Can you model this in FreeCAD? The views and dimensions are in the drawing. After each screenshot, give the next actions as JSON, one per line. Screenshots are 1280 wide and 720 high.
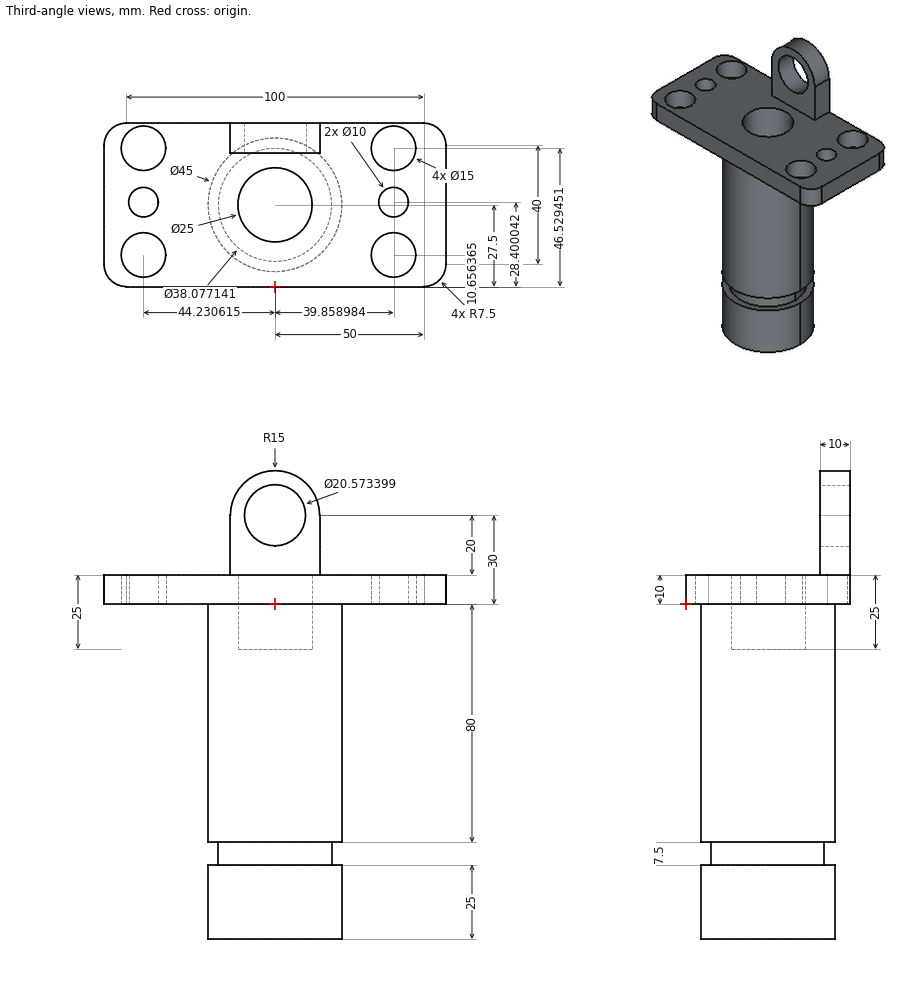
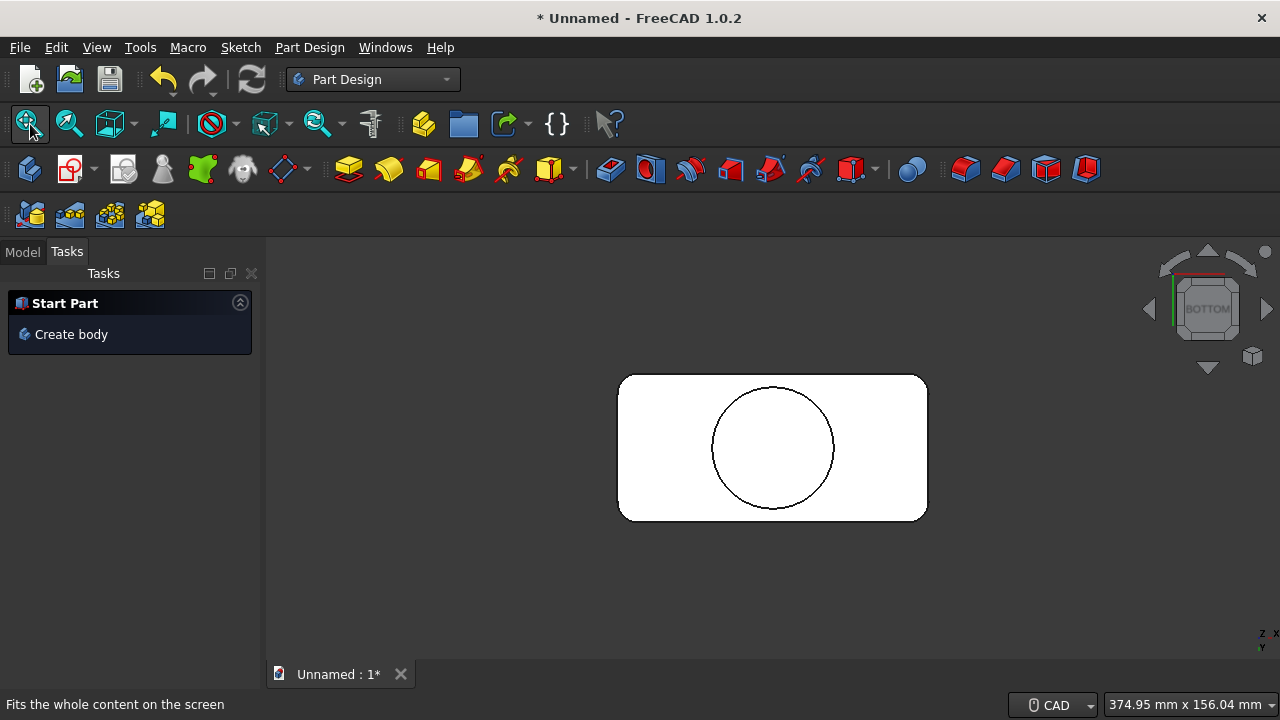
{"action": "left_click", "coordinate": [773, 447]}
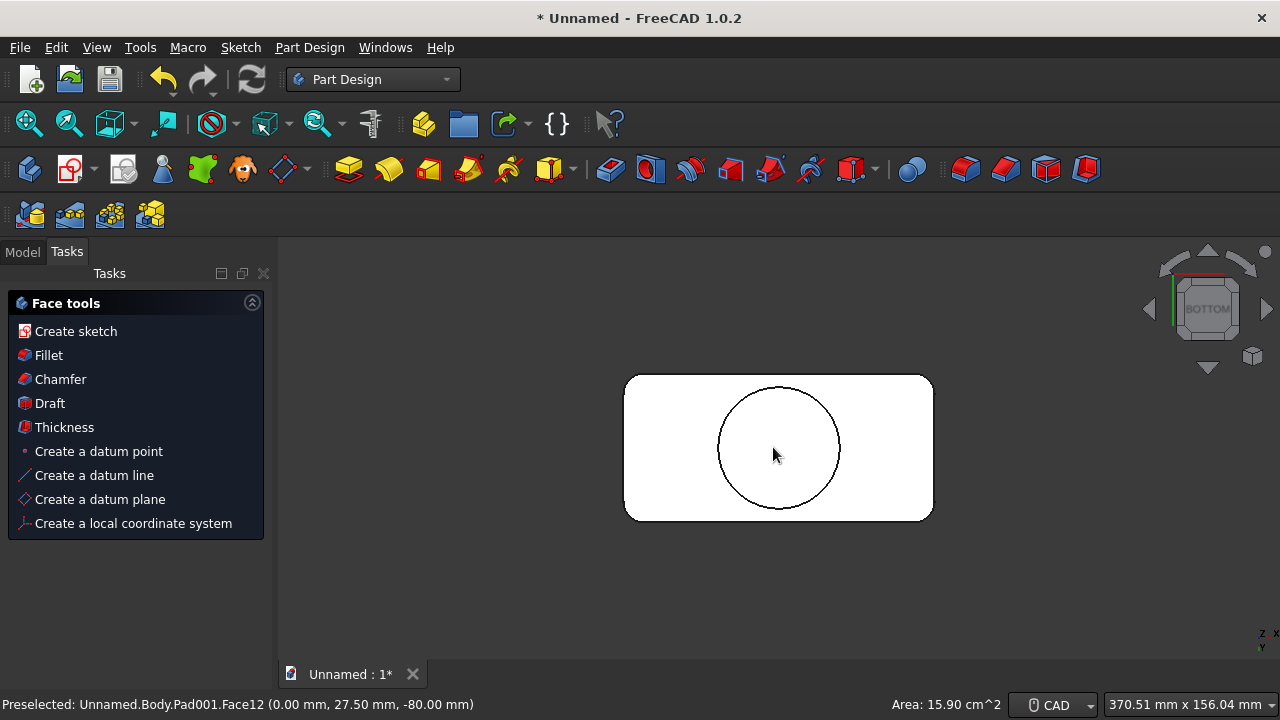
{"action": "left_click", "coordinate": [70, 170]}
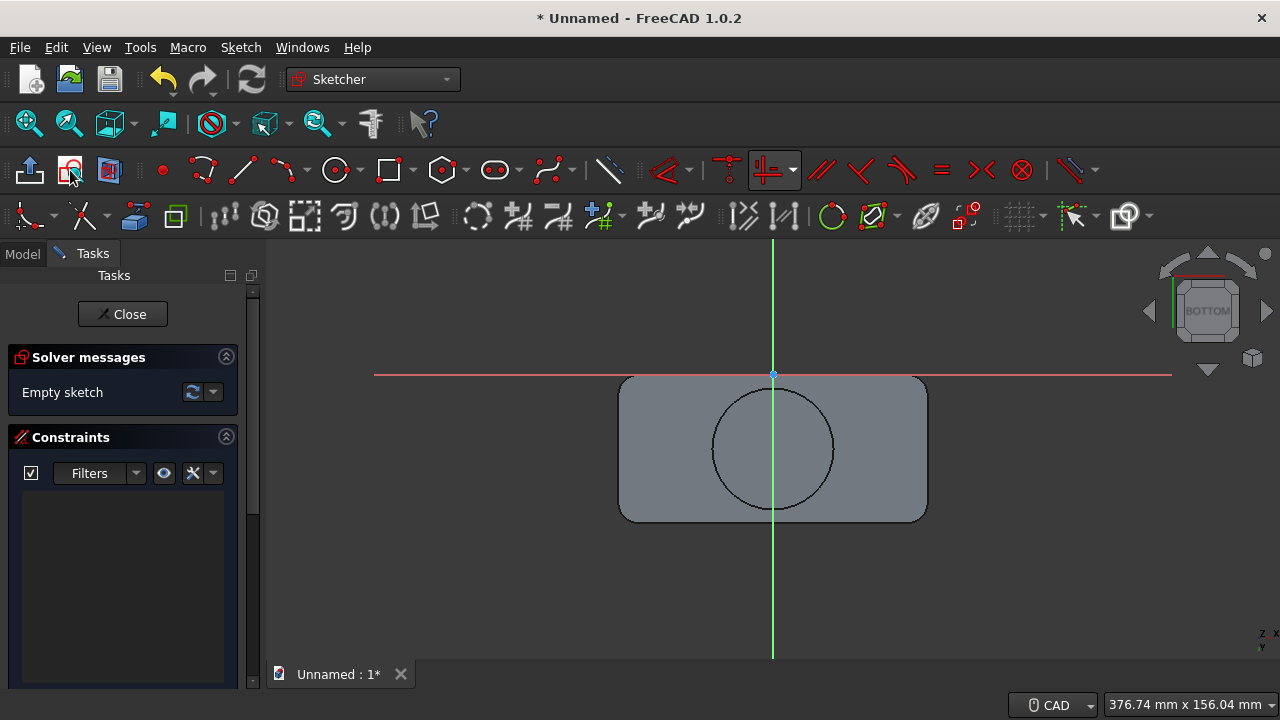
{"action": "scroll", "coordinate": [829, 428], "scroll_direction": "up", "scroll_amount": 4}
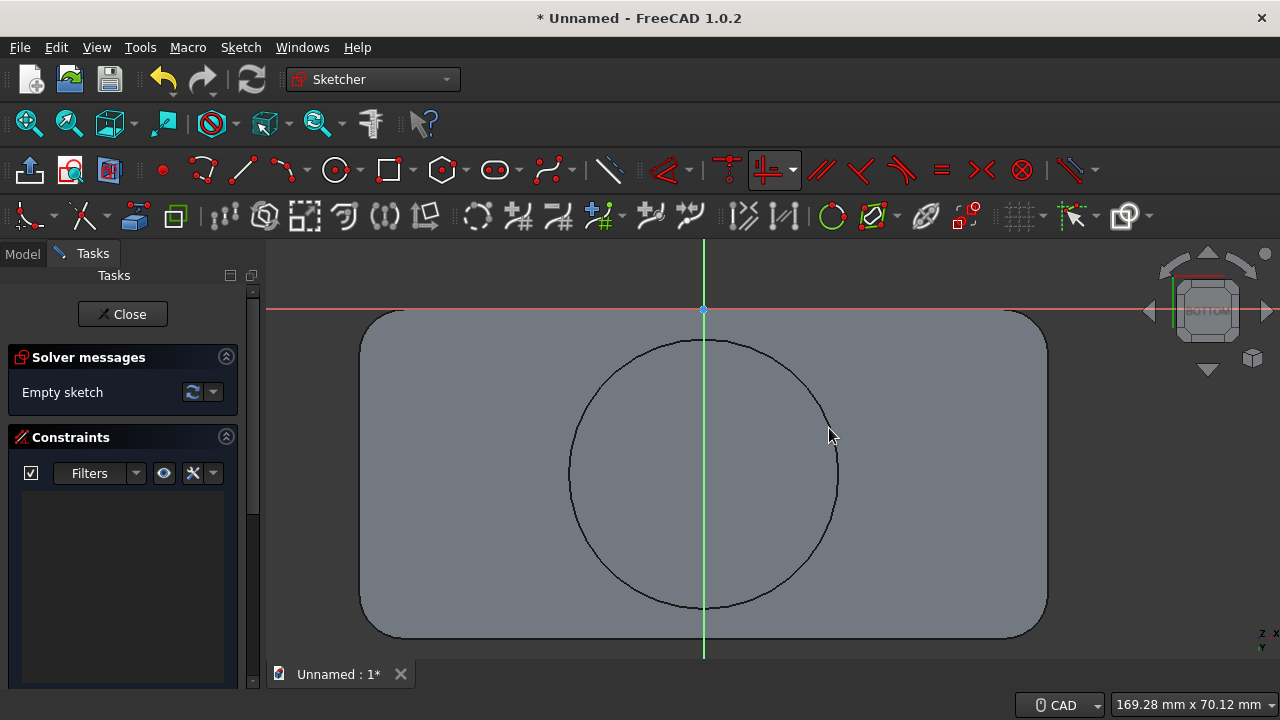
{"action": "left_click", "coordinate": [336, 170]}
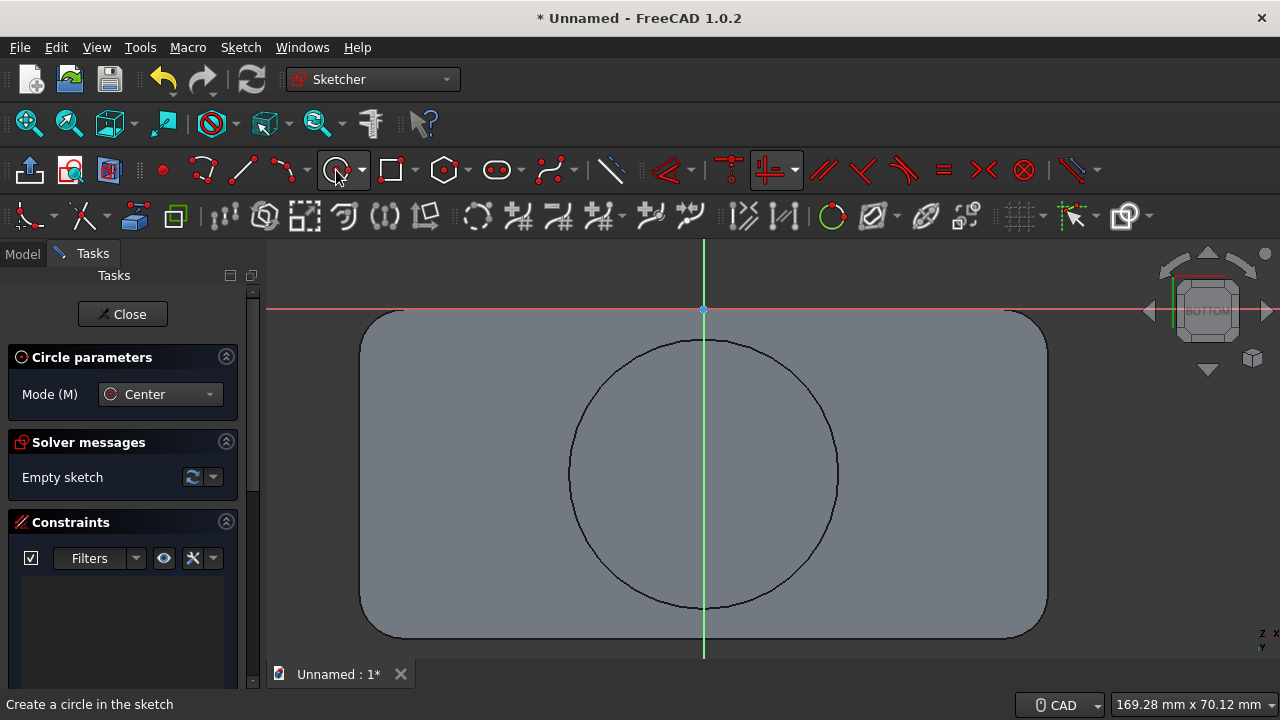
{"action": "left_click", "coordinate": [704, 474]}
{"action": "left_click", "coordinate": [784, 394]}
{"action": "key", "text": "Escape"}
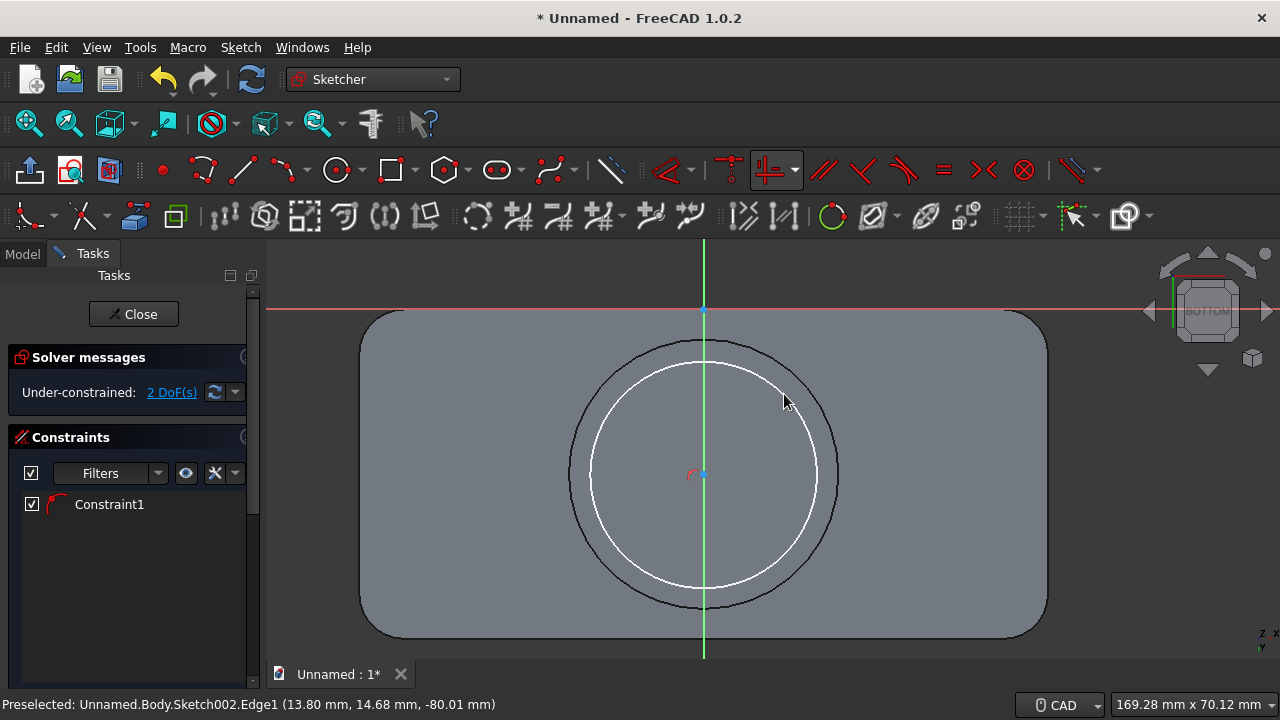
{"action": "left_click", "coordinate": [666, 170]}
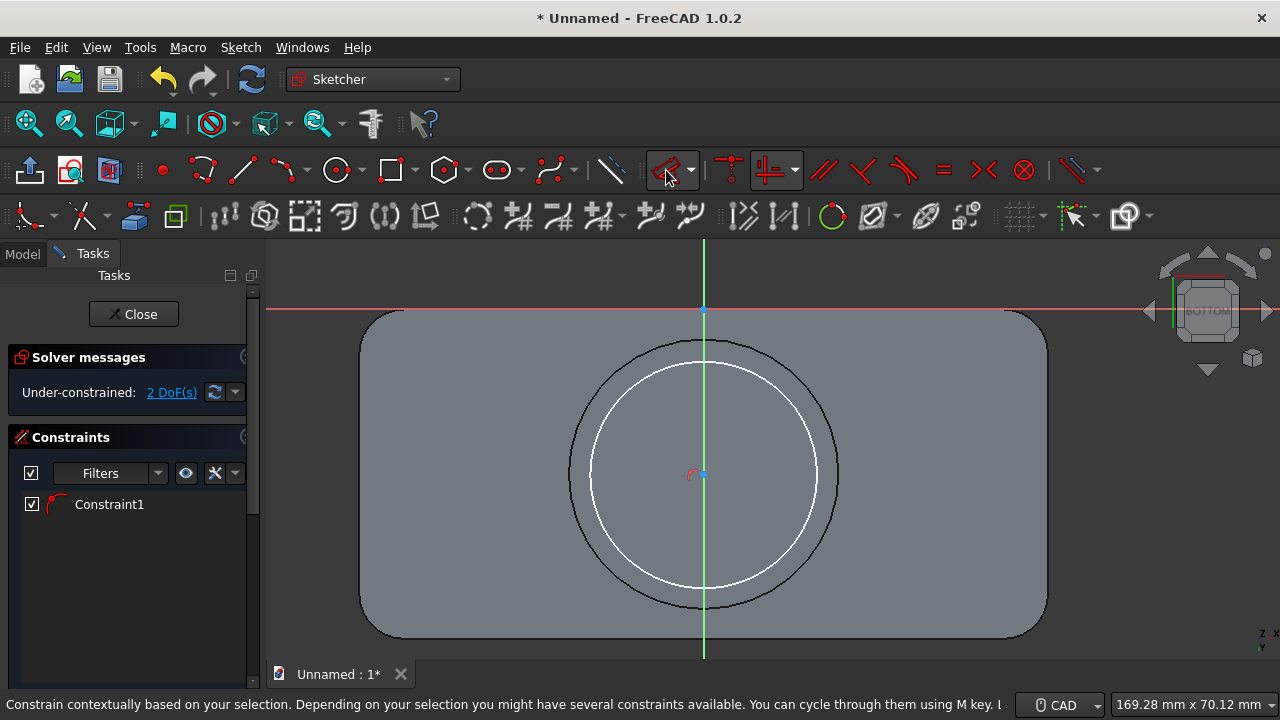
{"action": "left_click", "coordinate": [784, 395]}
{"action": "left_click", "coordinate": [807, 372]}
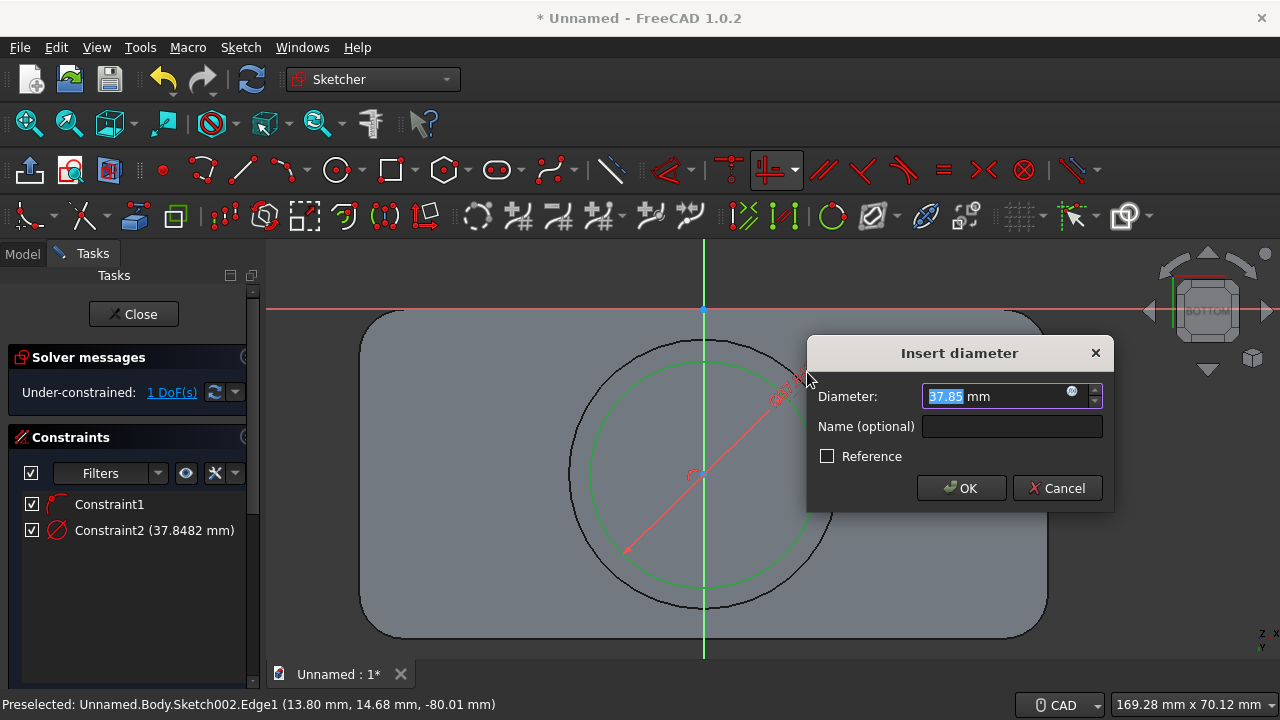
{"action": "type", "text": "38.077141"}
{"action": "key", "text": "Return"}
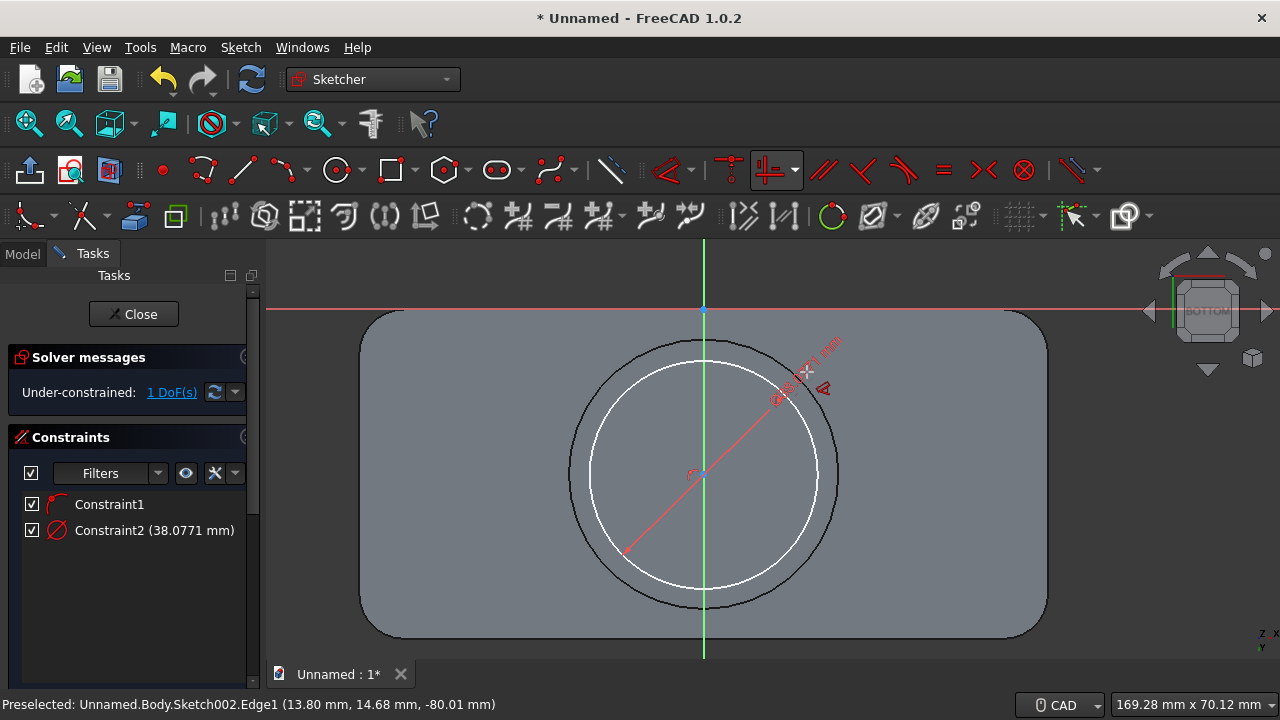
{"action": "left_click", "coordinate": [704, 475]}
{"action": "left_click", "coordinate": [738, 430]}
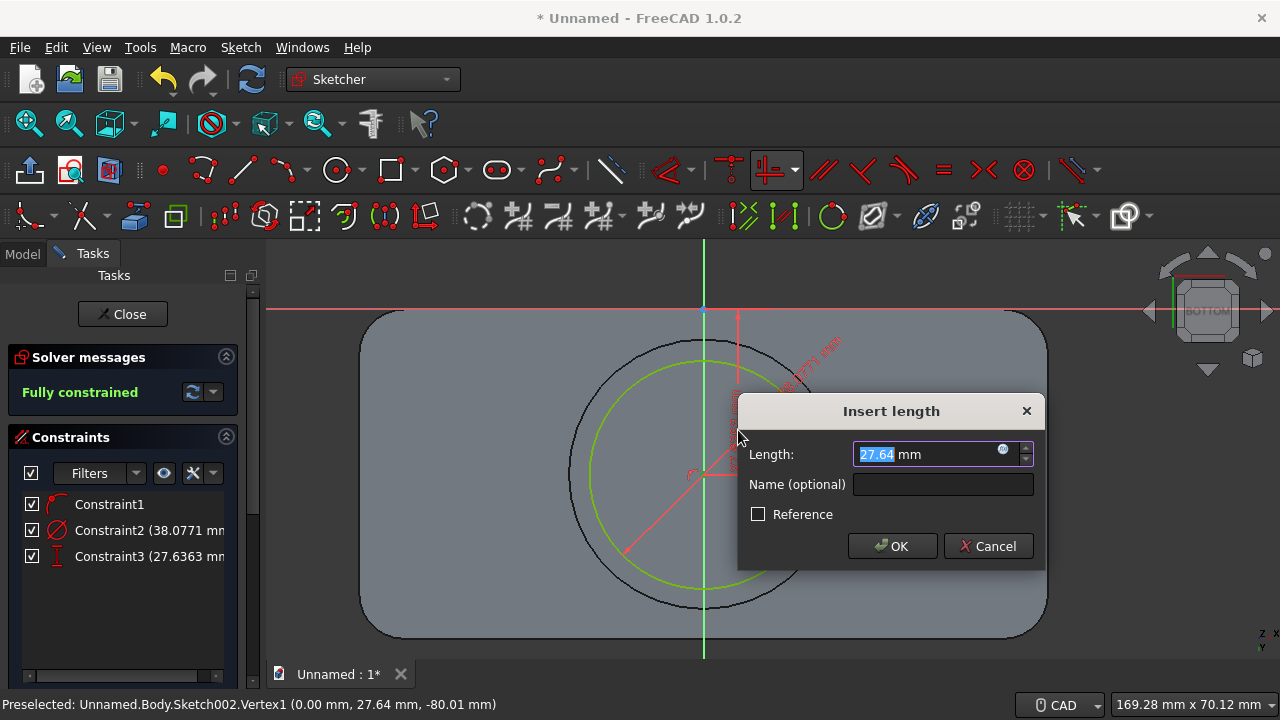
{"action": "type", "text": "27.5"}
{"action": "key", "text": "Return"}
{"action": "key", "text": "Escape"}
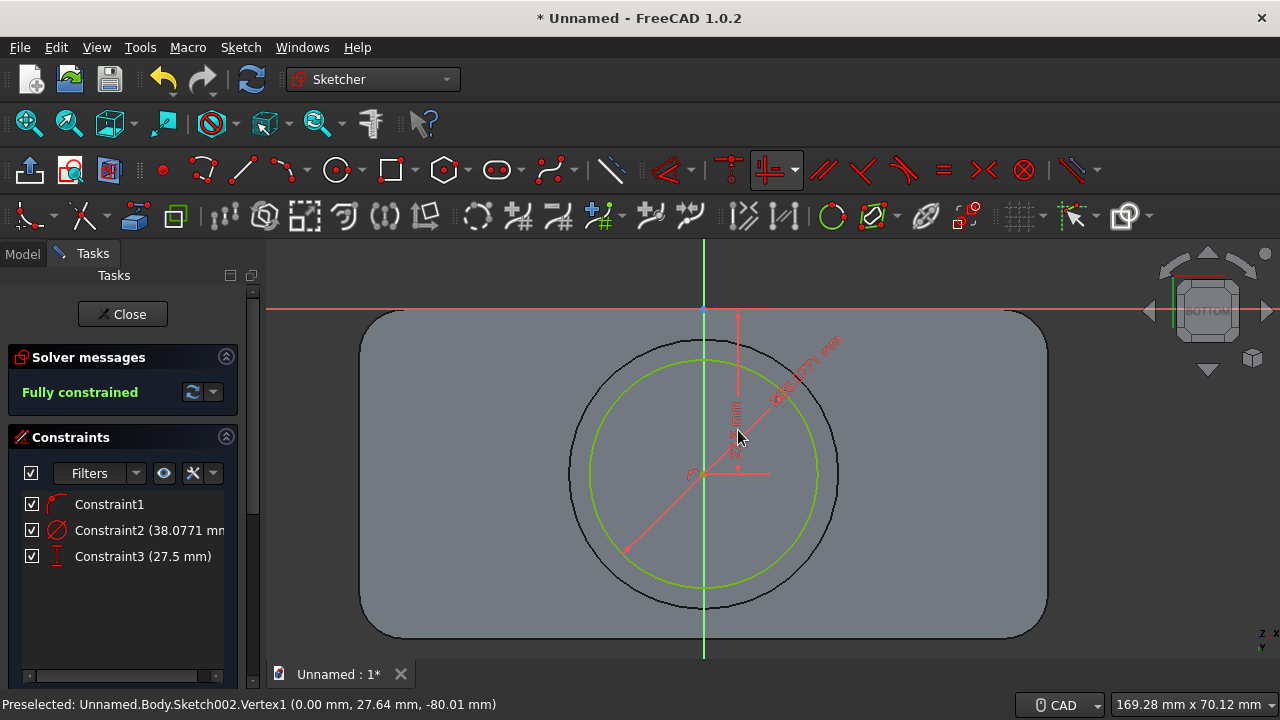
{"action": "left_click", "coordinate": [123, 314]}